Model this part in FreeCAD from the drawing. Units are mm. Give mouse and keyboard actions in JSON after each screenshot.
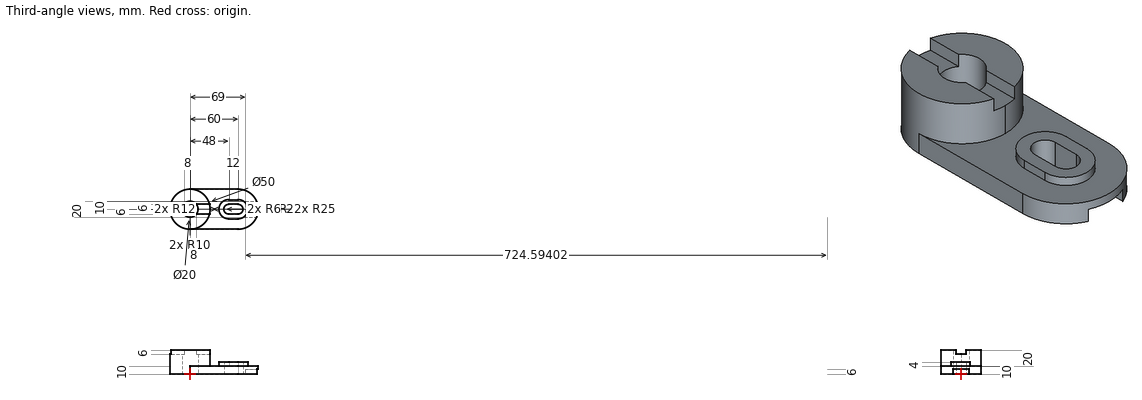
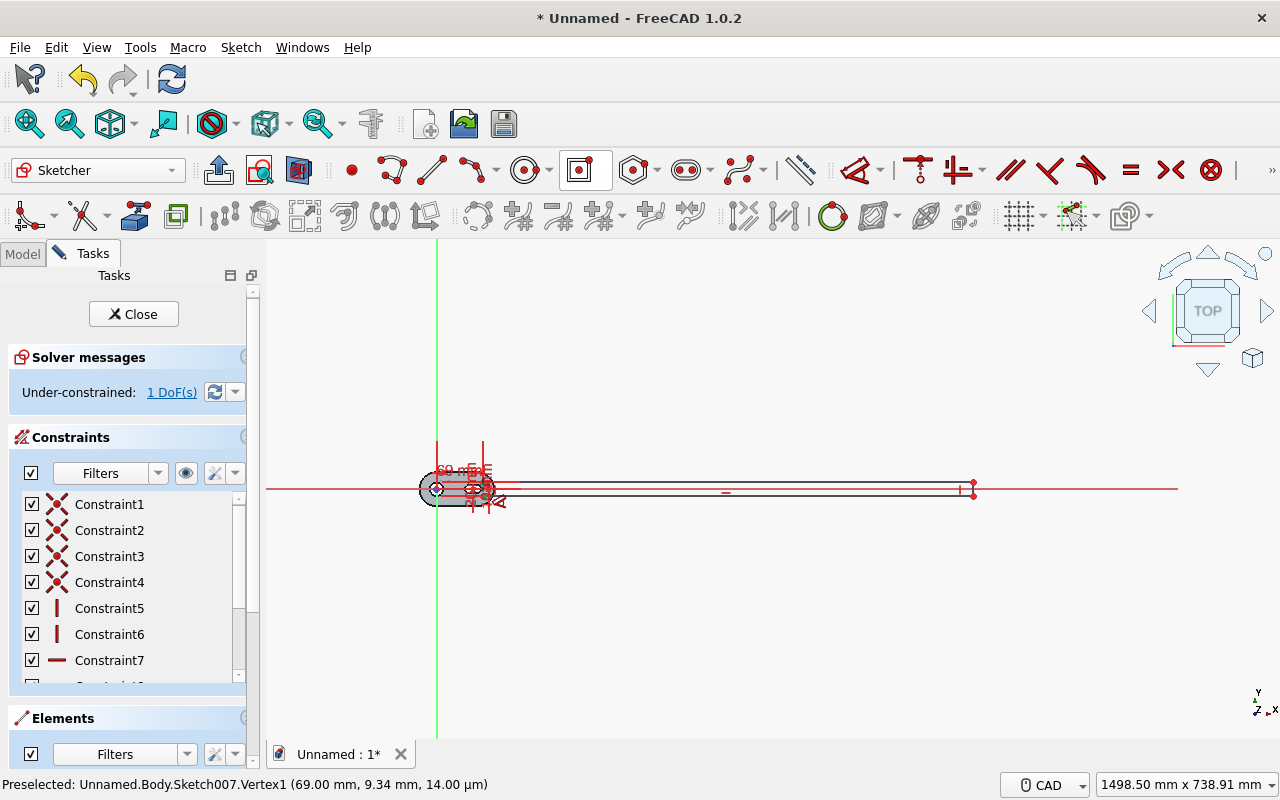
{"action": "scroll", "coordinate": [581, 496], "scroll_direction": "up", "scroll_amount": 4}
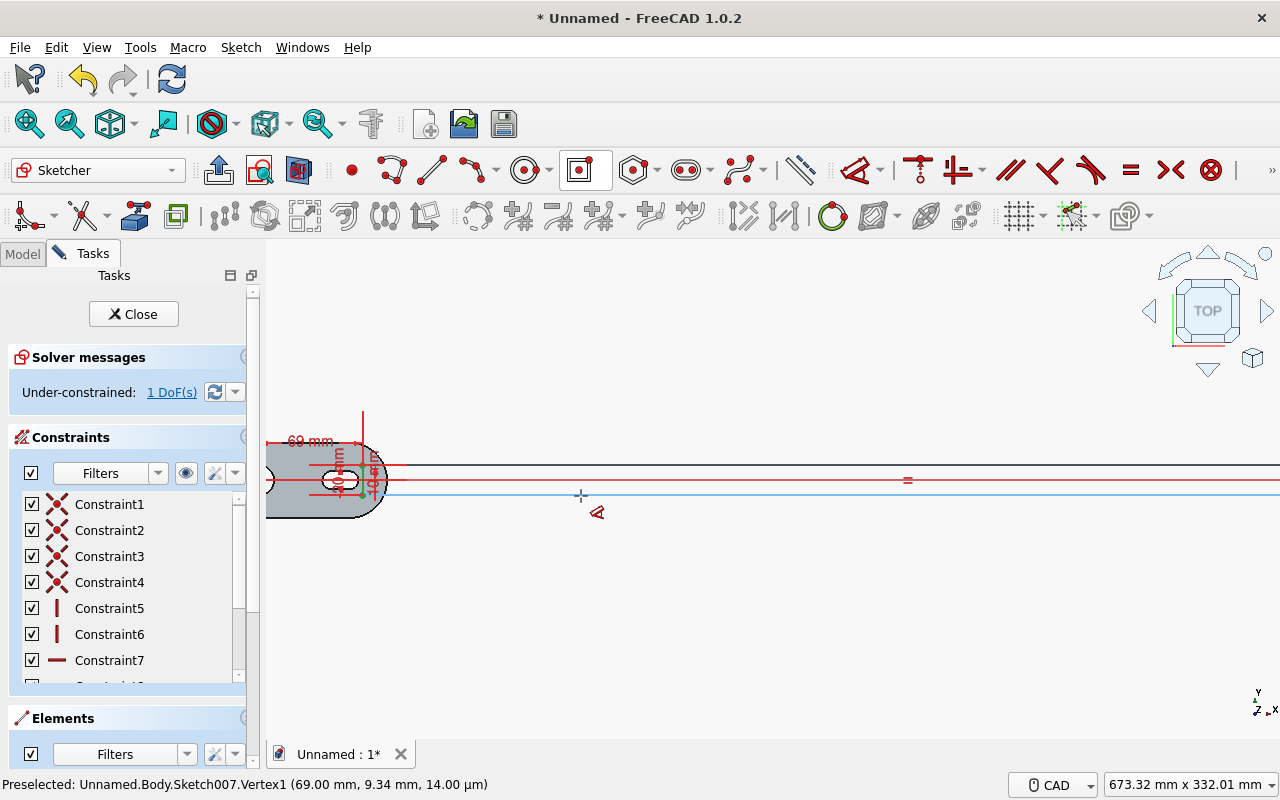
{"action": "left_click", "coordinate": [581, 495]}
{"action": "left_click", "coordinate": [739, 529]}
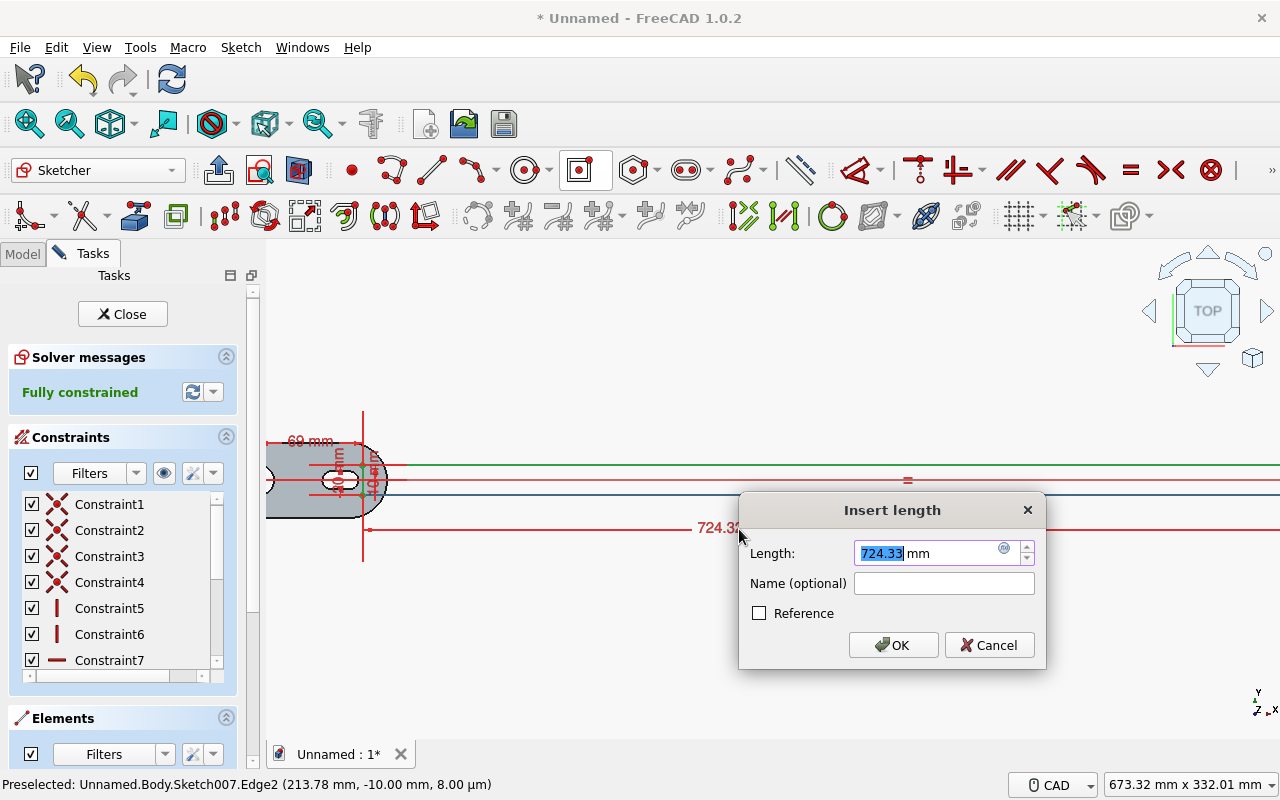
{"action": "type", "text": "724.59402"}
{"action": "key", "text": "Return"}
{"action": "key", "text": "Escape"}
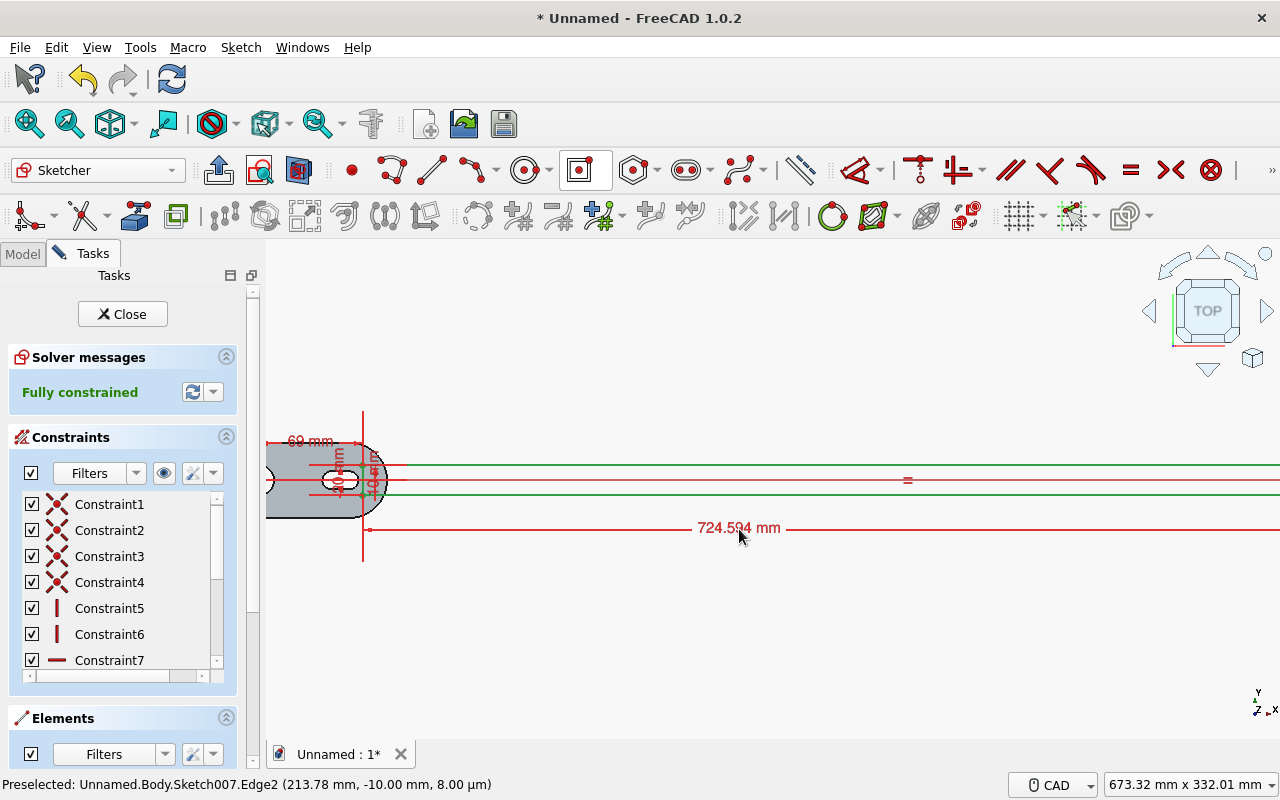
{"action": "left_click", "coordinate": [123, 314]}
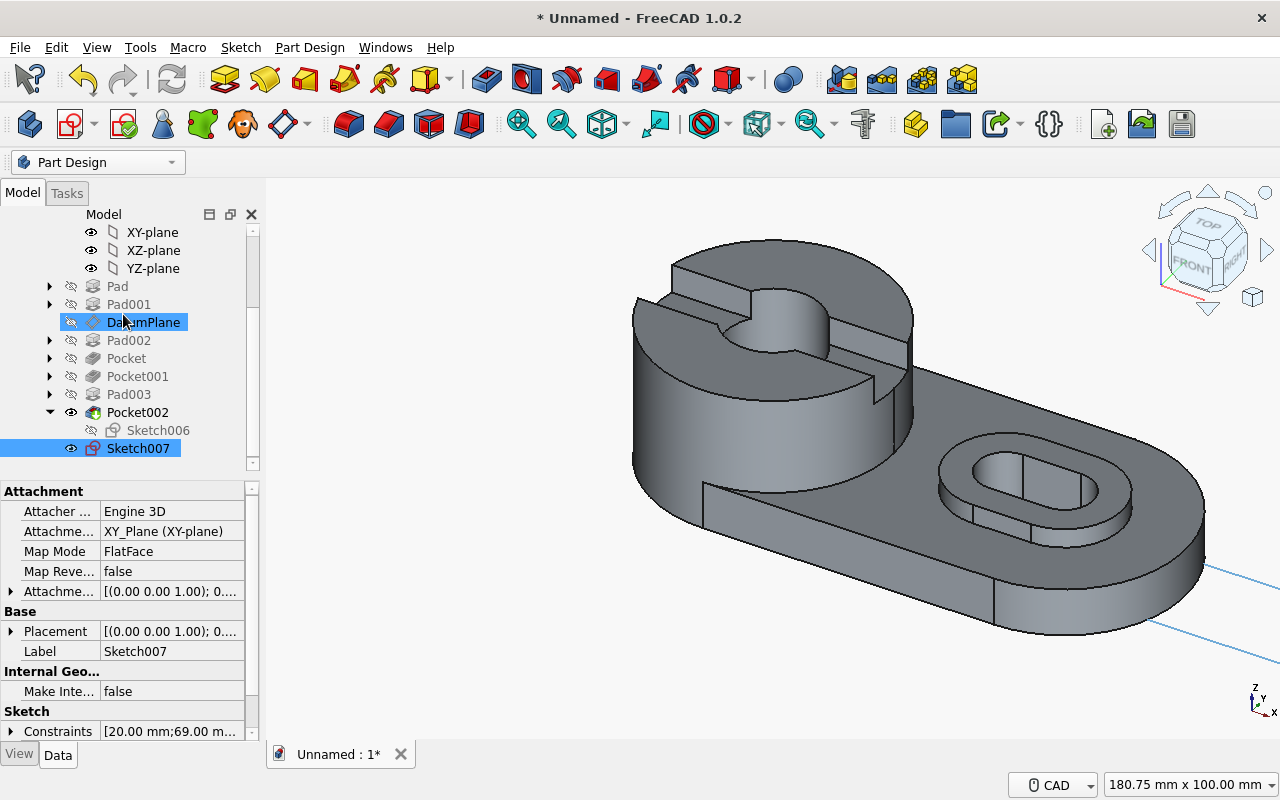
{"action": "left_click", "coordinate": [488, 80]}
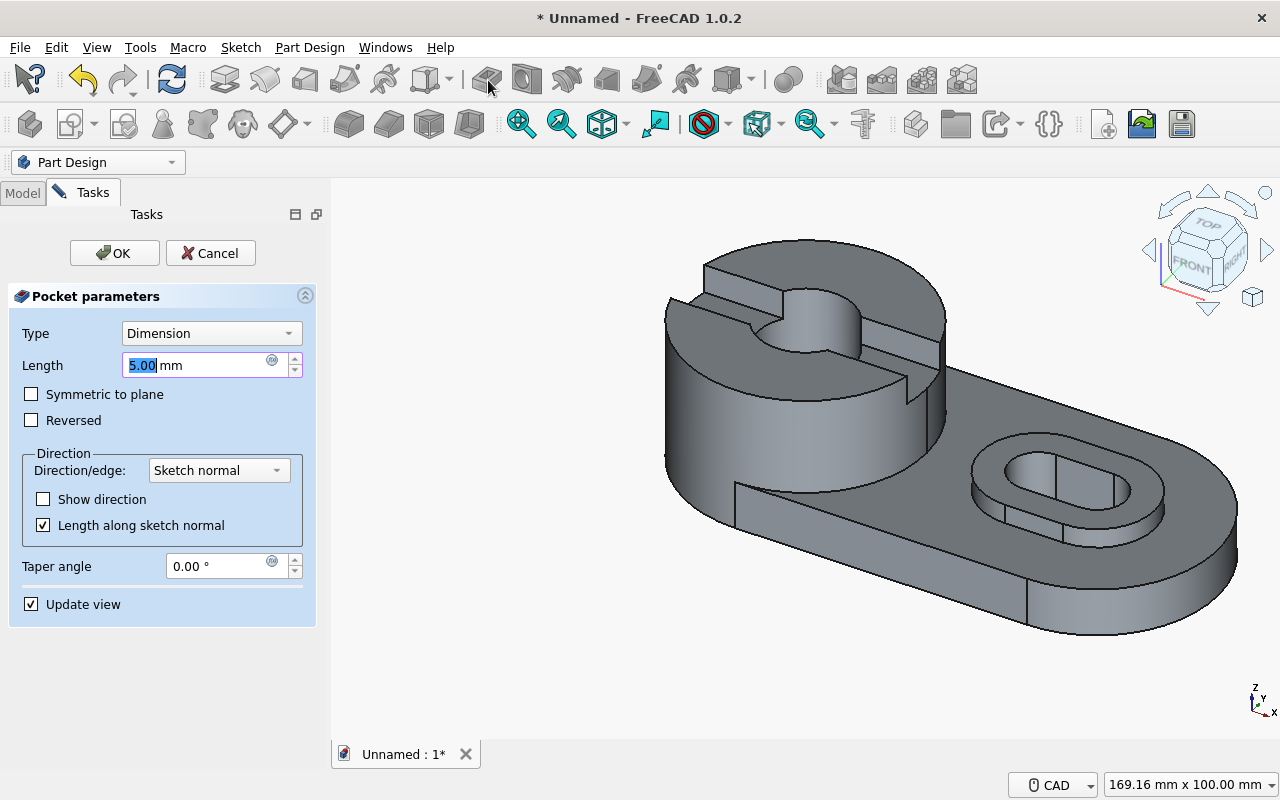
{"action": "left_click", "coordinate": [212, 334]}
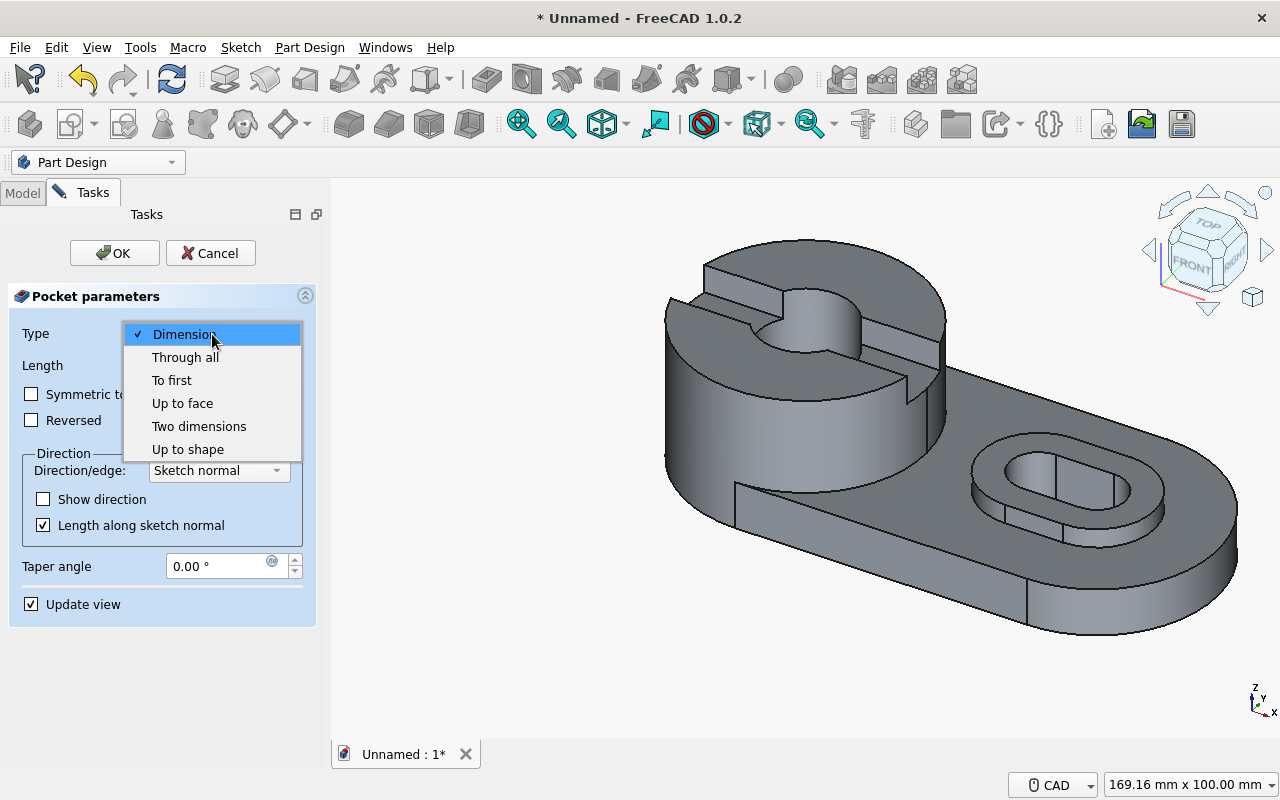
{"action": "left_click", "coordinate": [212, 426]}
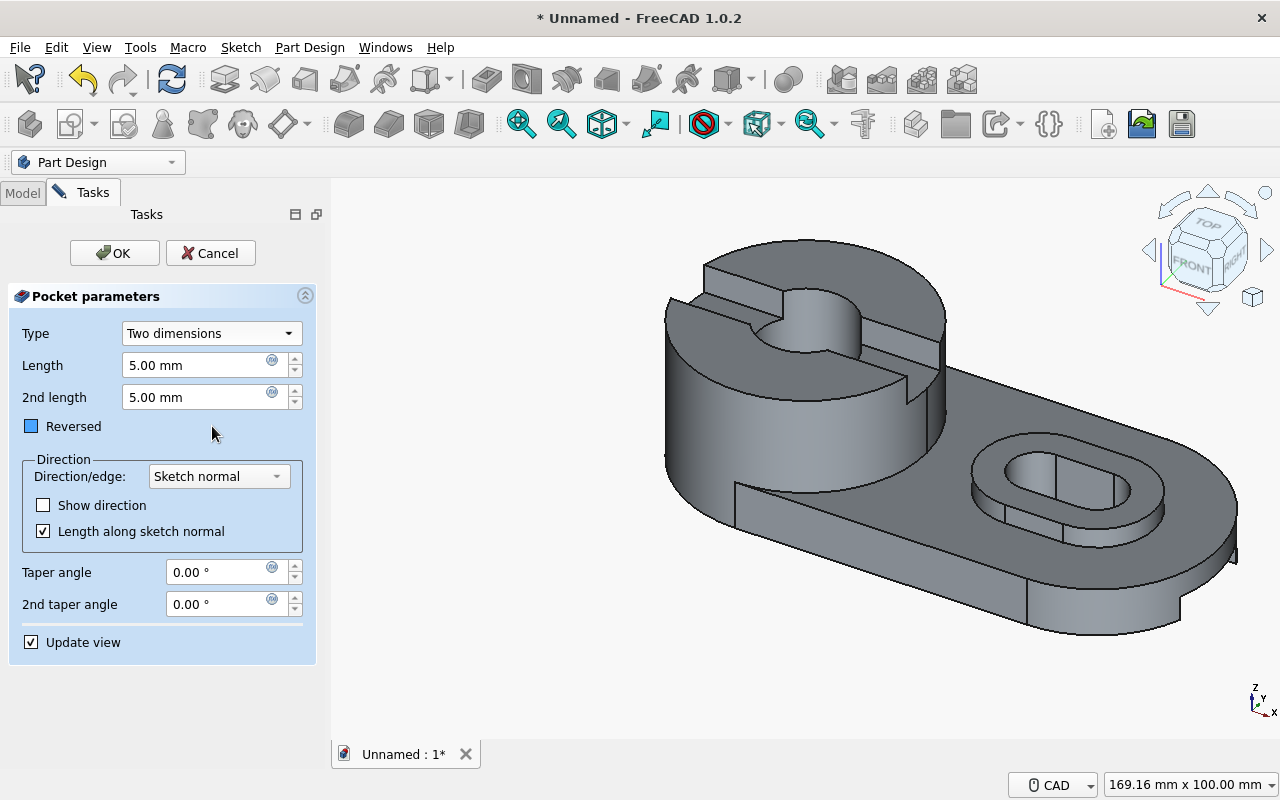
{"action": "triple_click", "coordinate": [204, 365]}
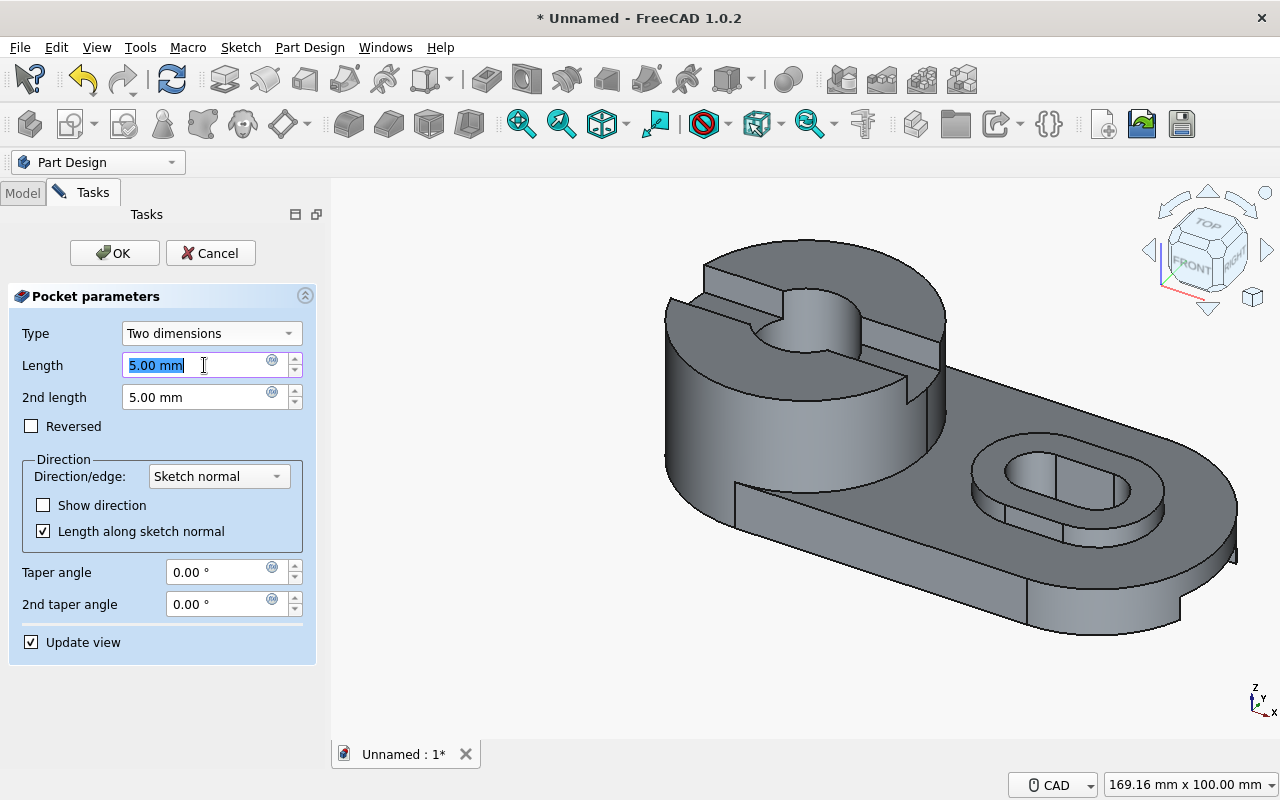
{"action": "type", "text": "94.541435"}
{"action": "key", "text": "Tab"}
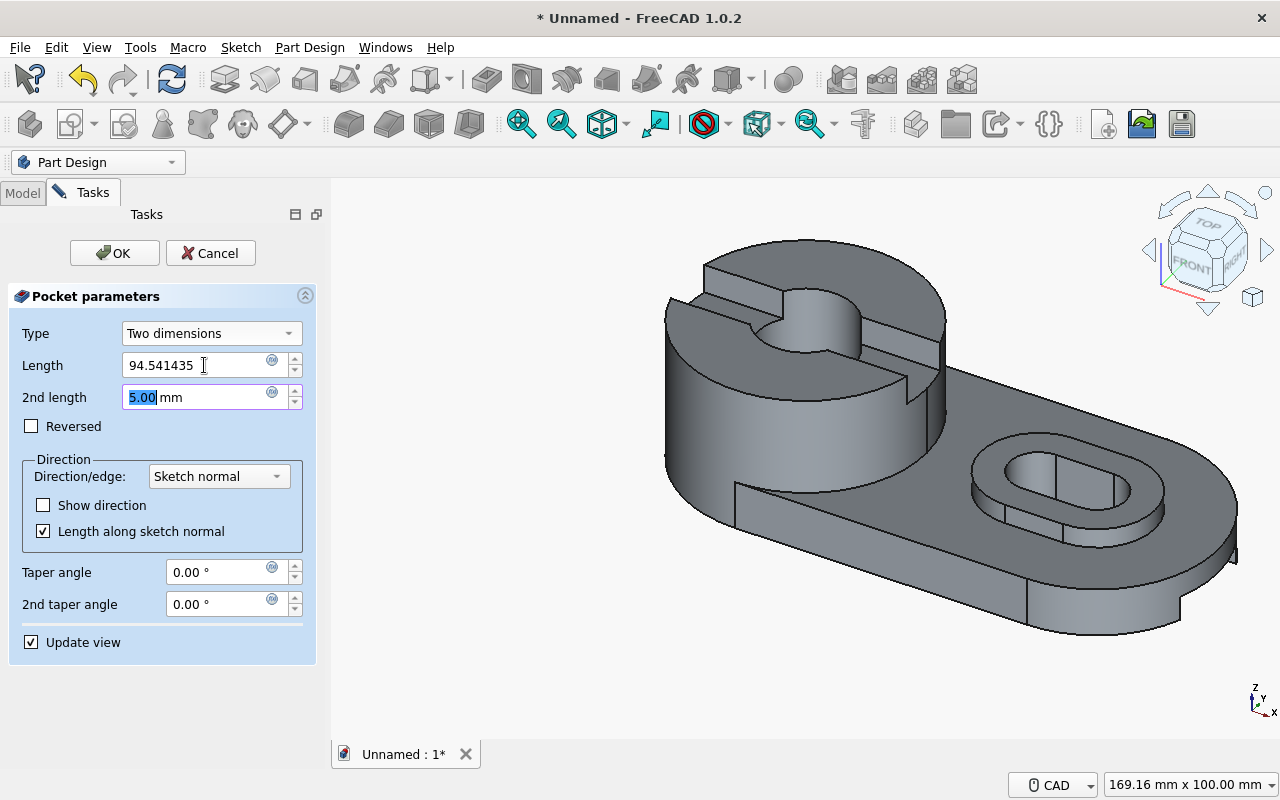
{"action": "type", "text": "6"}
{"action": "key", "text": "Tab"}